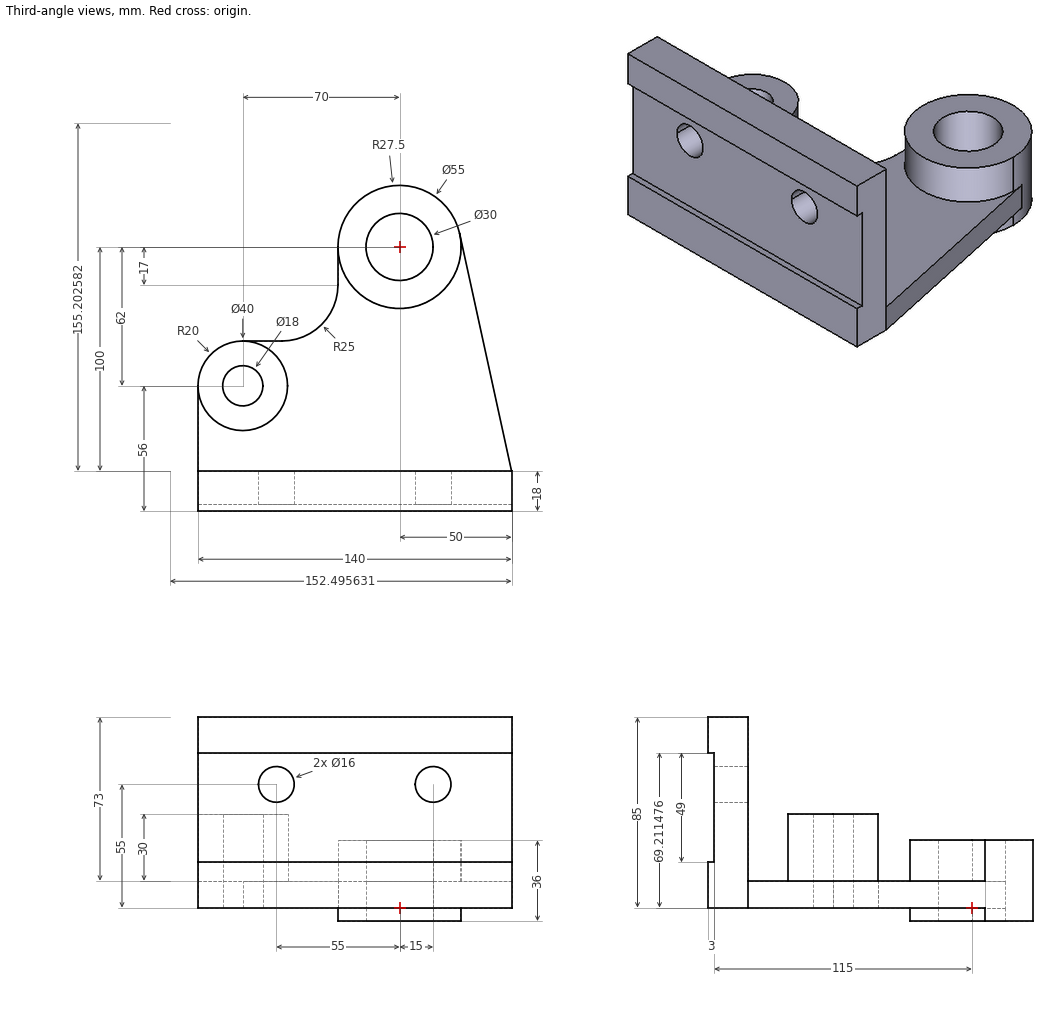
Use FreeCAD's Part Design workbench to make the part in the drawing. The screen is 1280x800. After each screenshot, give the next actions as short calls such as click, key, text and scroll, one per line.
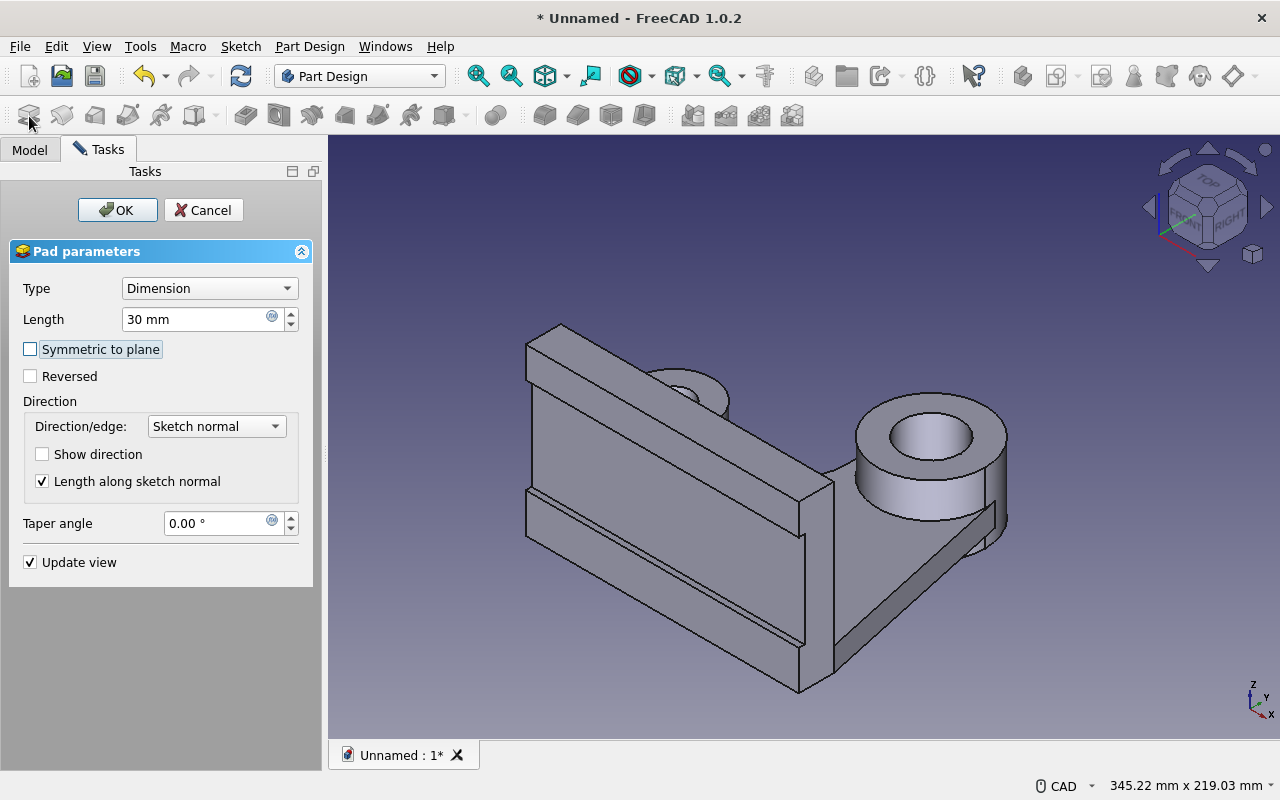
click(118, 210)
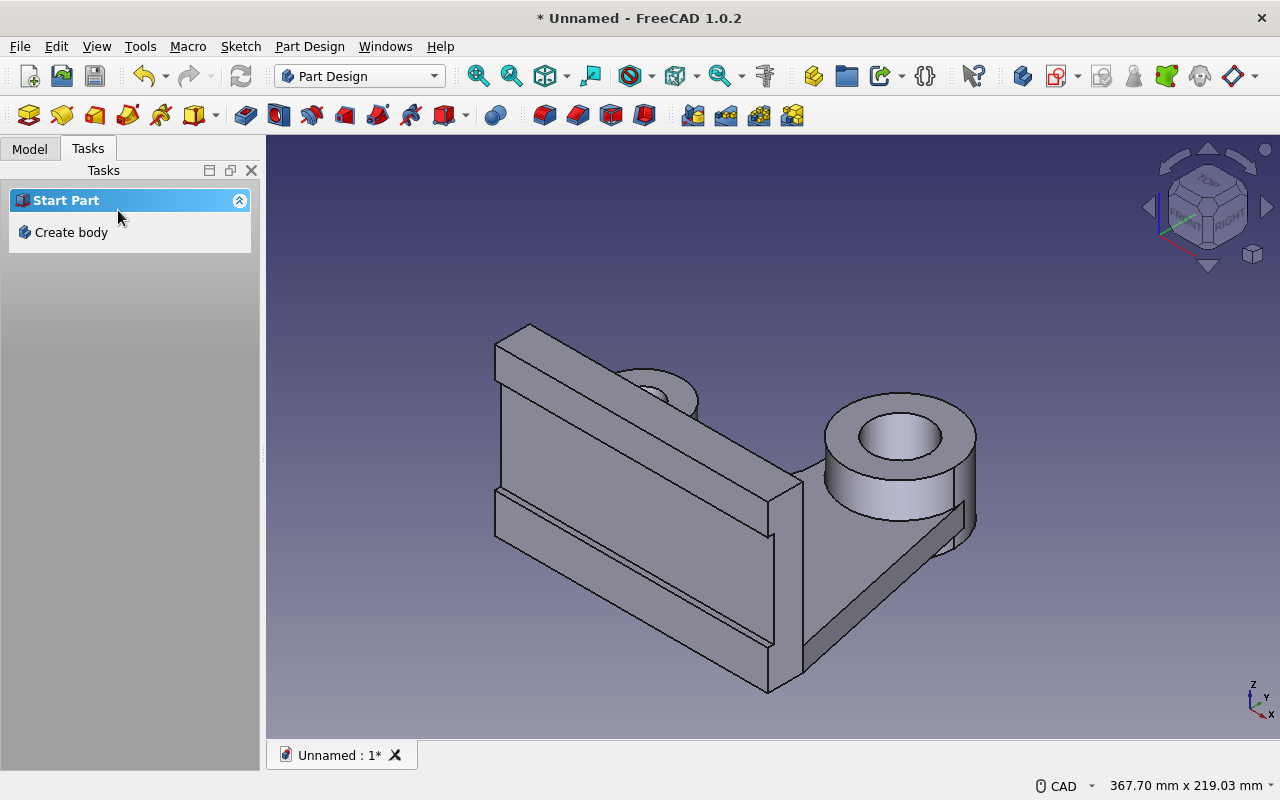
key(4)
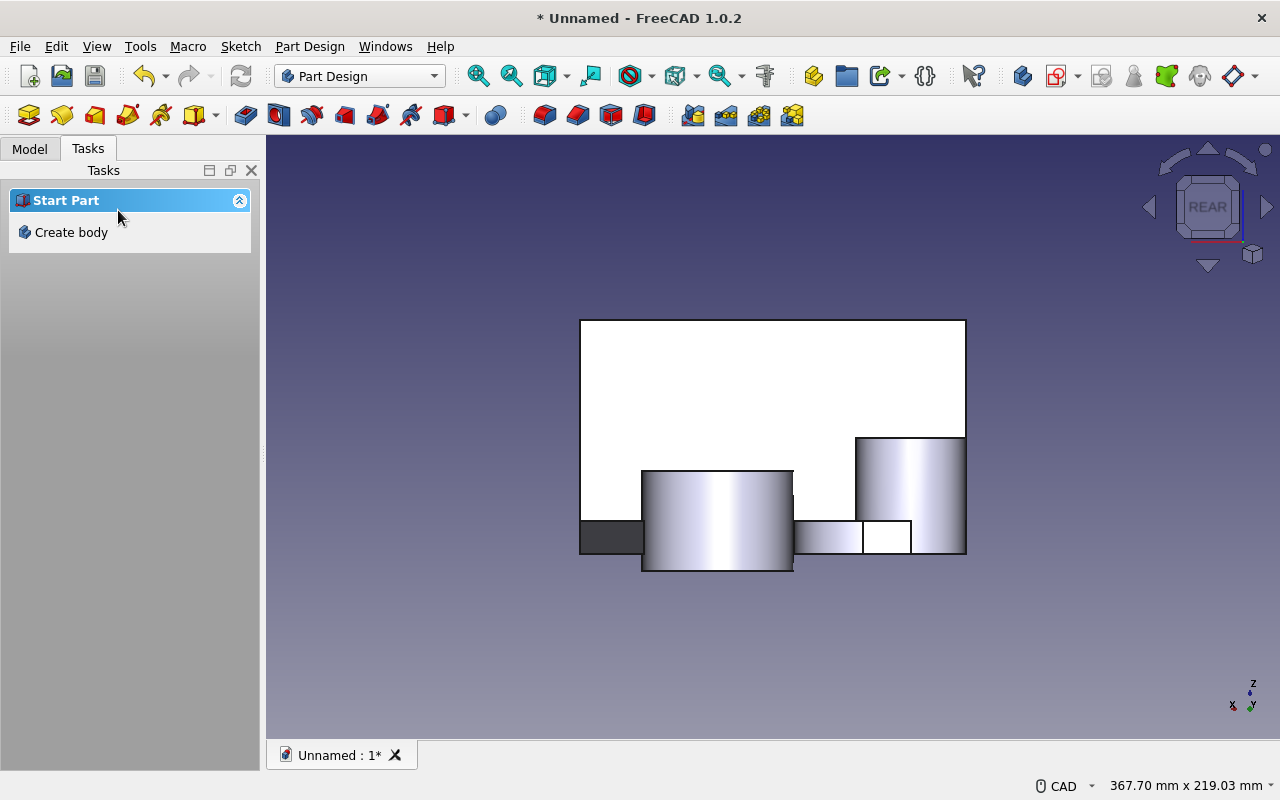
click(479, 76)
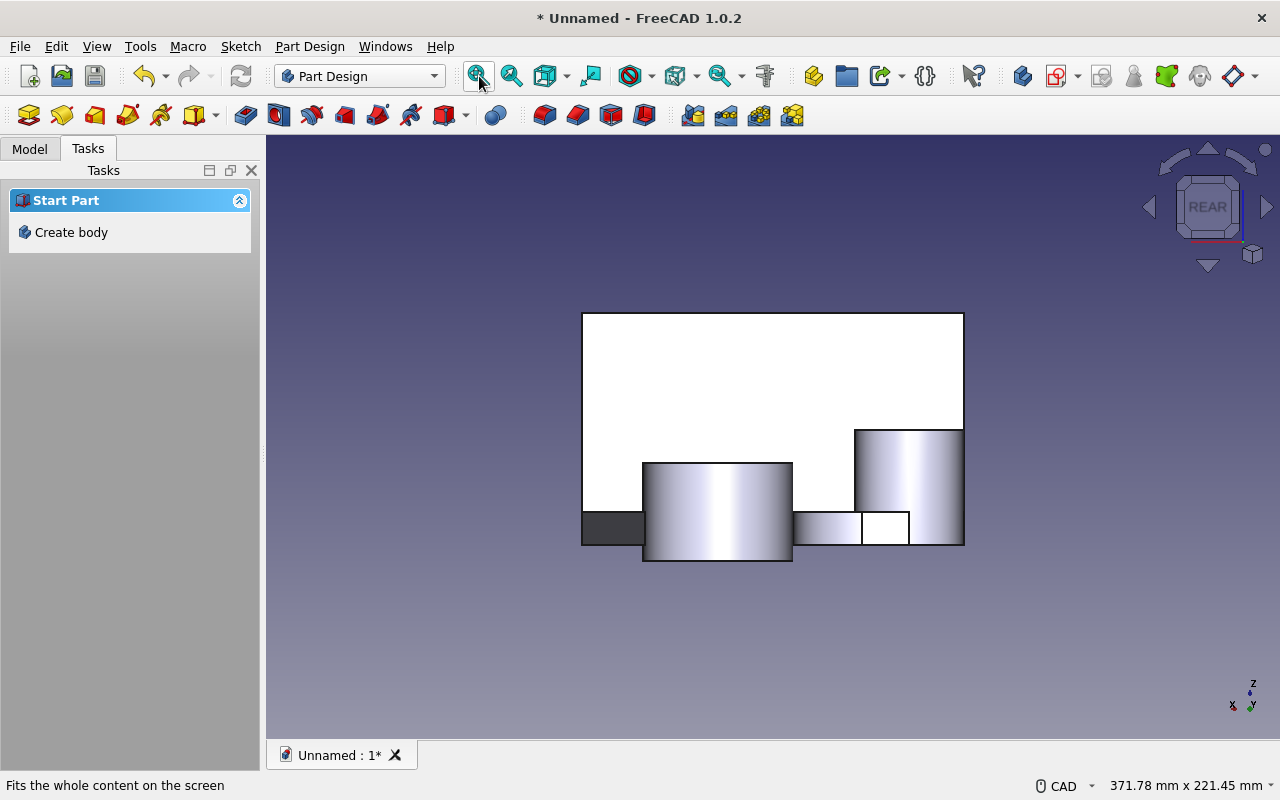
click(718, 411)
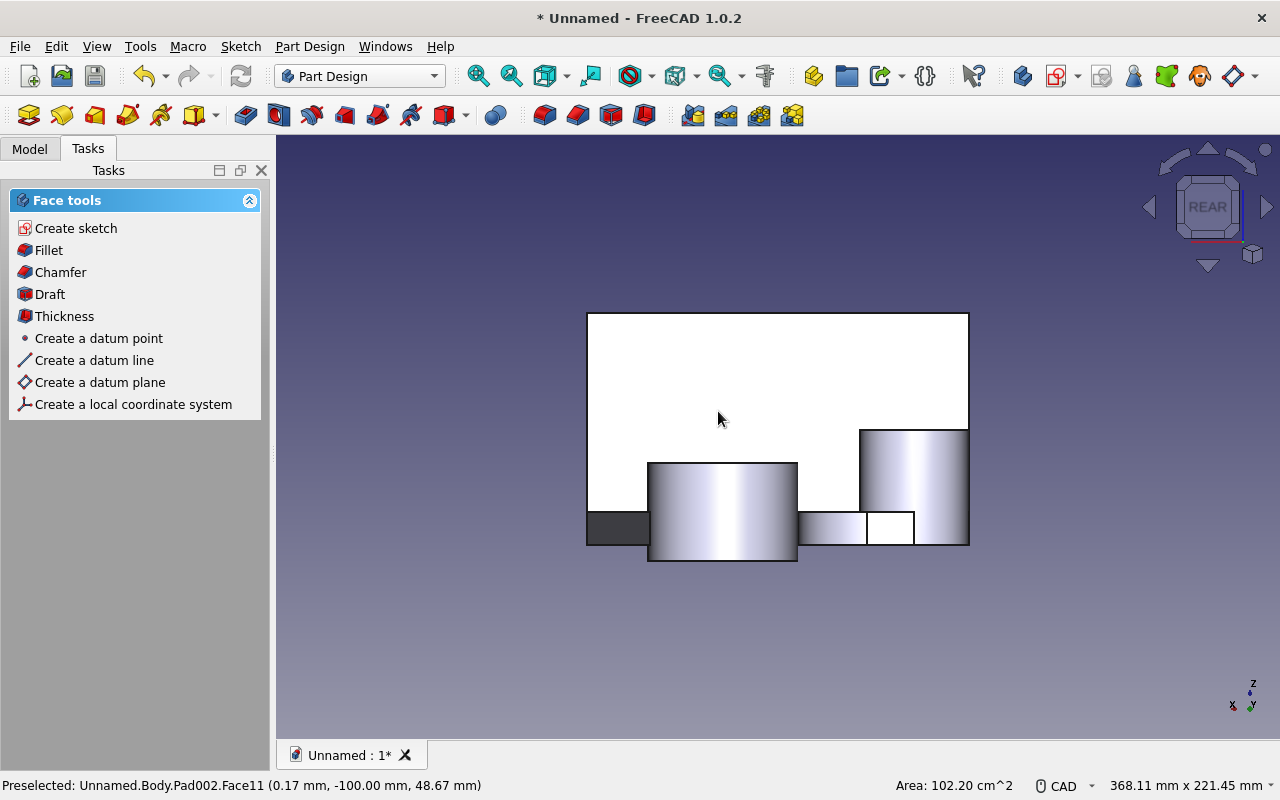
click(1056, 76)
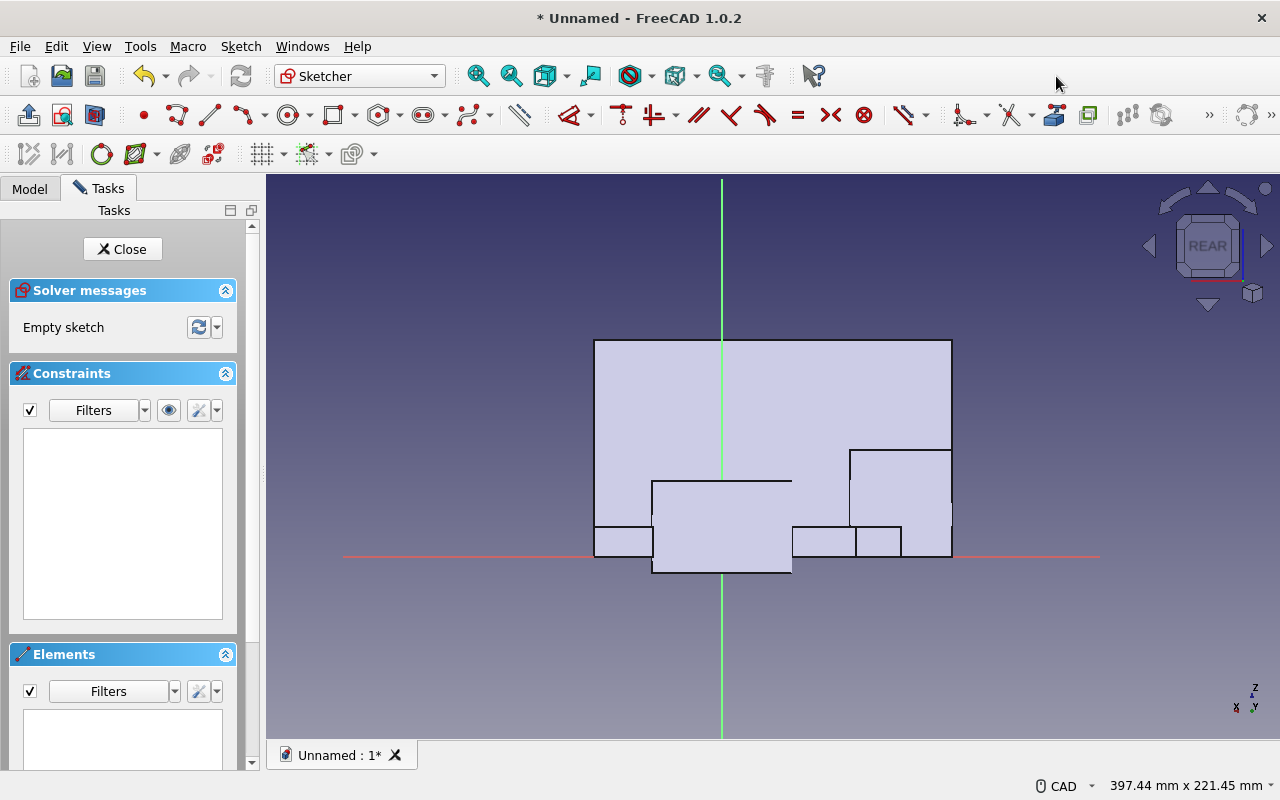
click(95, 116)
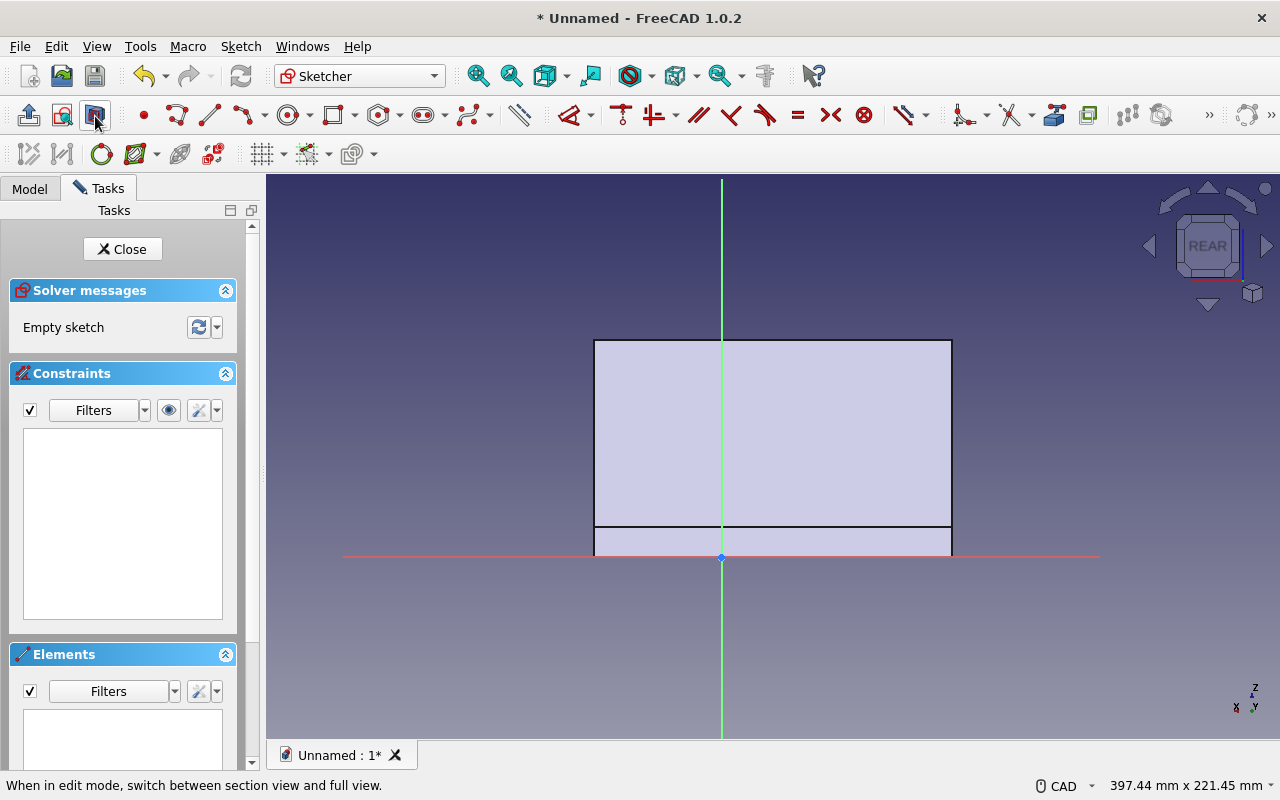
scroll(829, 494, up, 4)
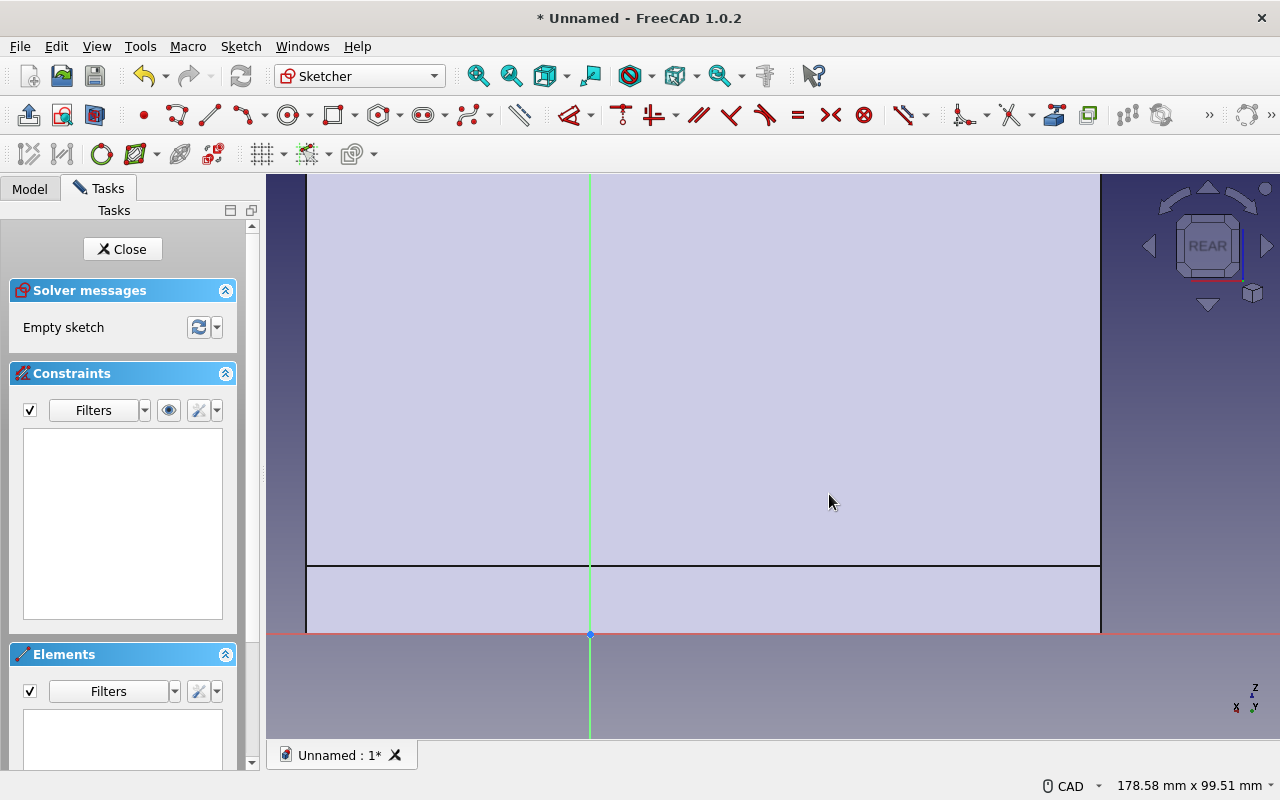
click(288, 116)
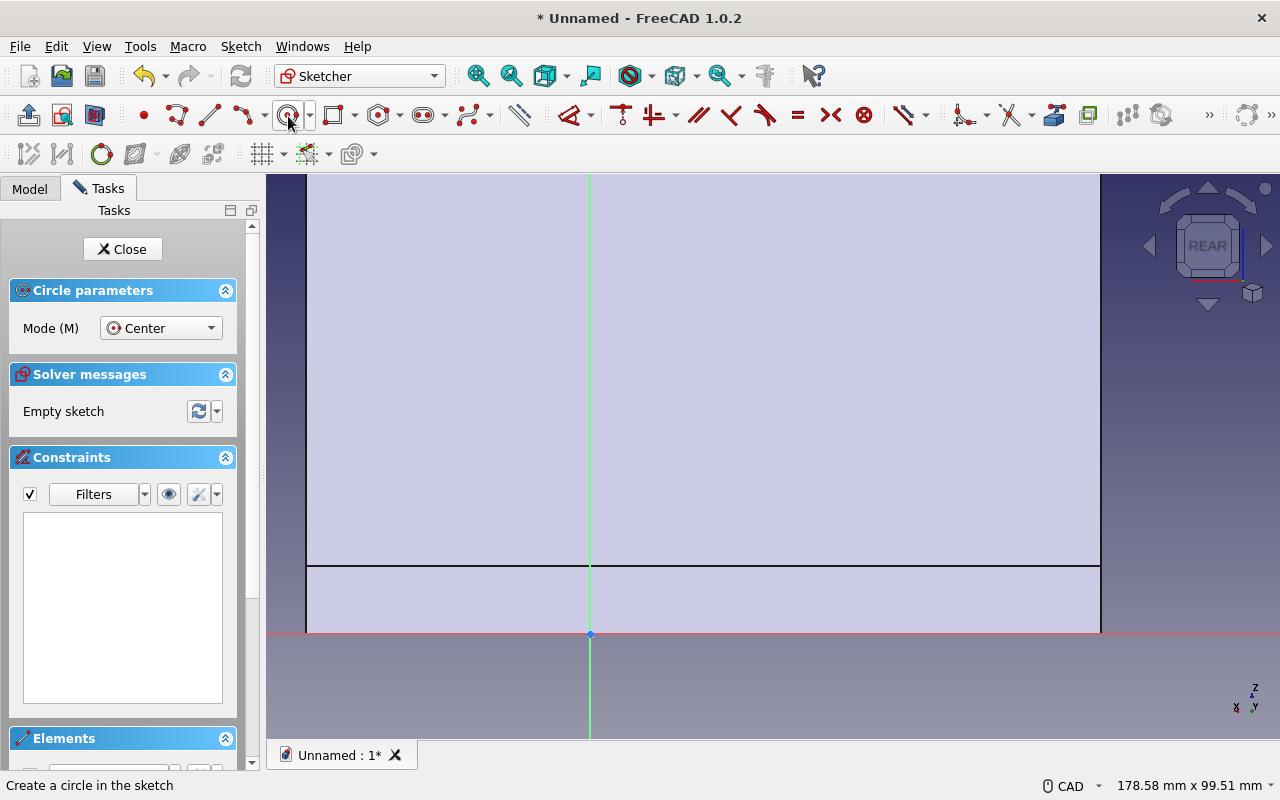
click(902, 322)
click(935, 290)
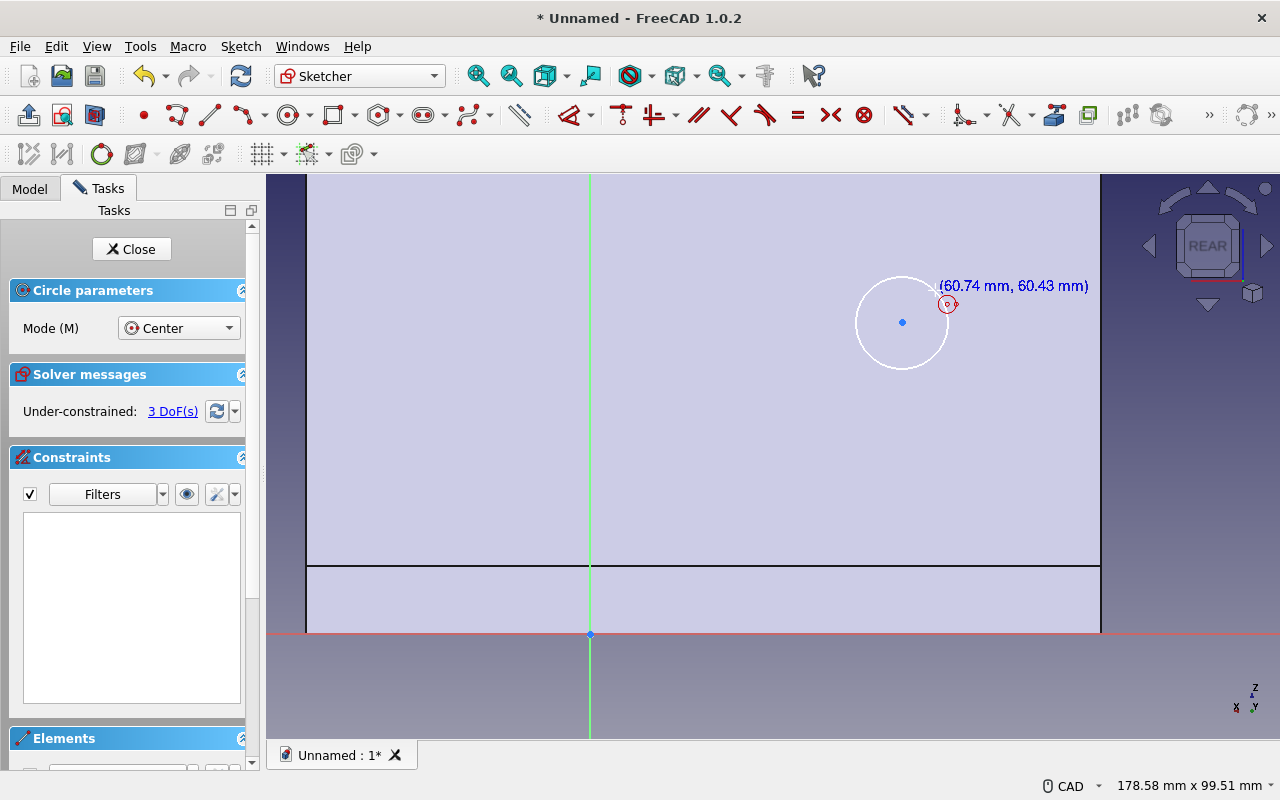
click(505, 322)
click(537, 290)
key(Escape)